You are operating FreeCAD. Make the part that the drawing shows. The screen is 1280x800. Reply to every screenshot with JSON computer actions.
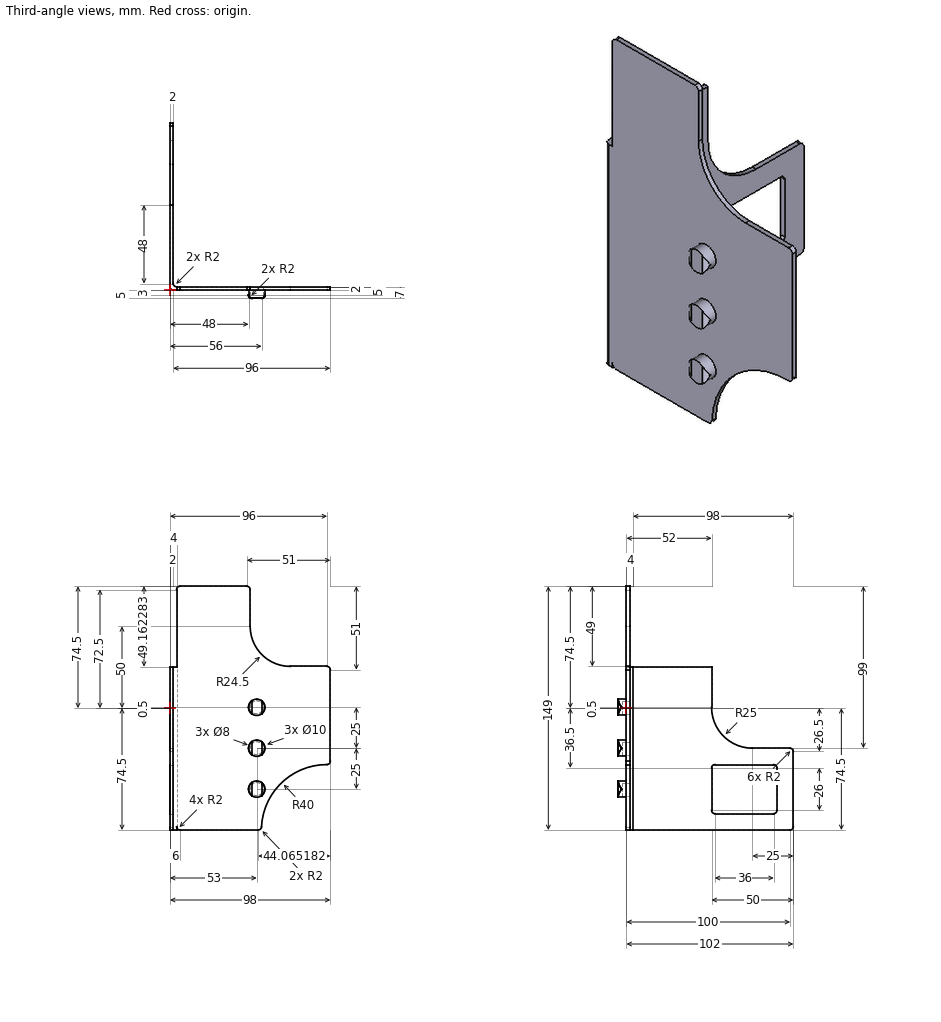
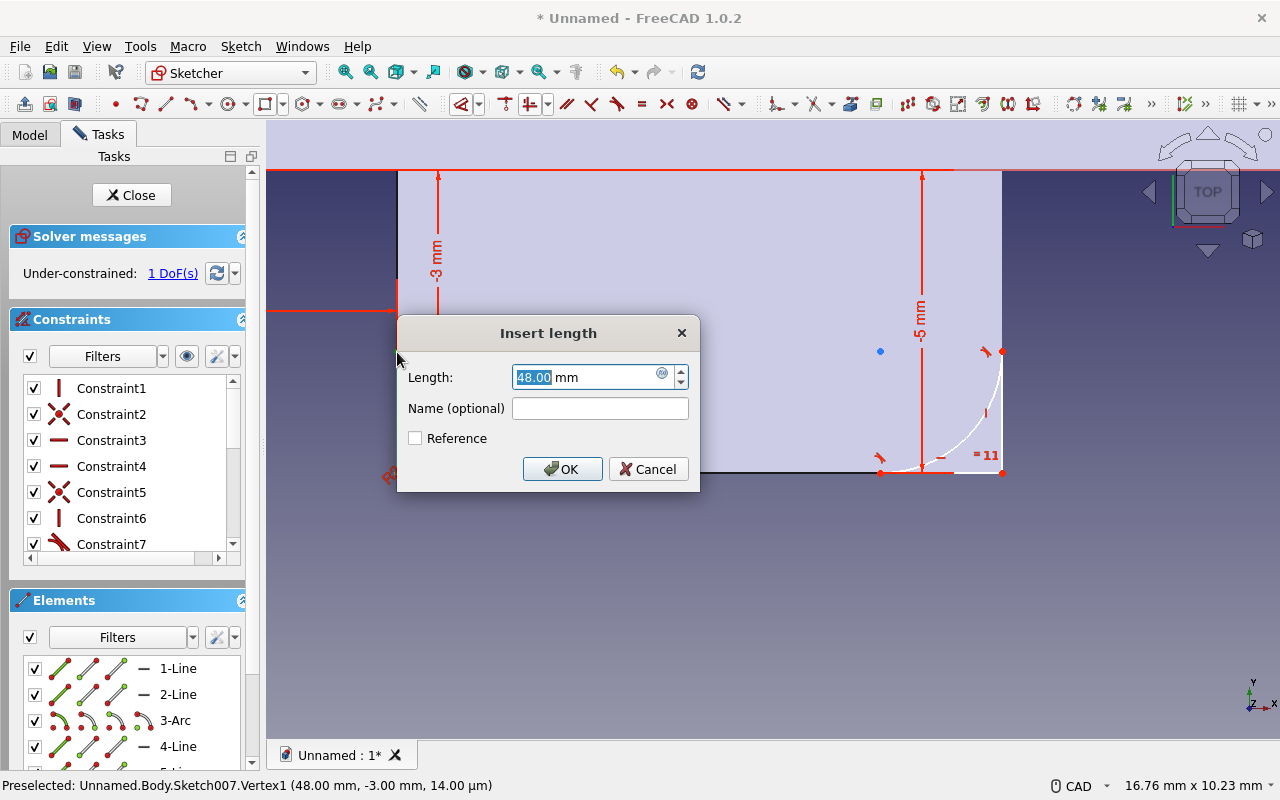
{"action": "type", "text": "48"}
{"action": "key", "text": "Return"}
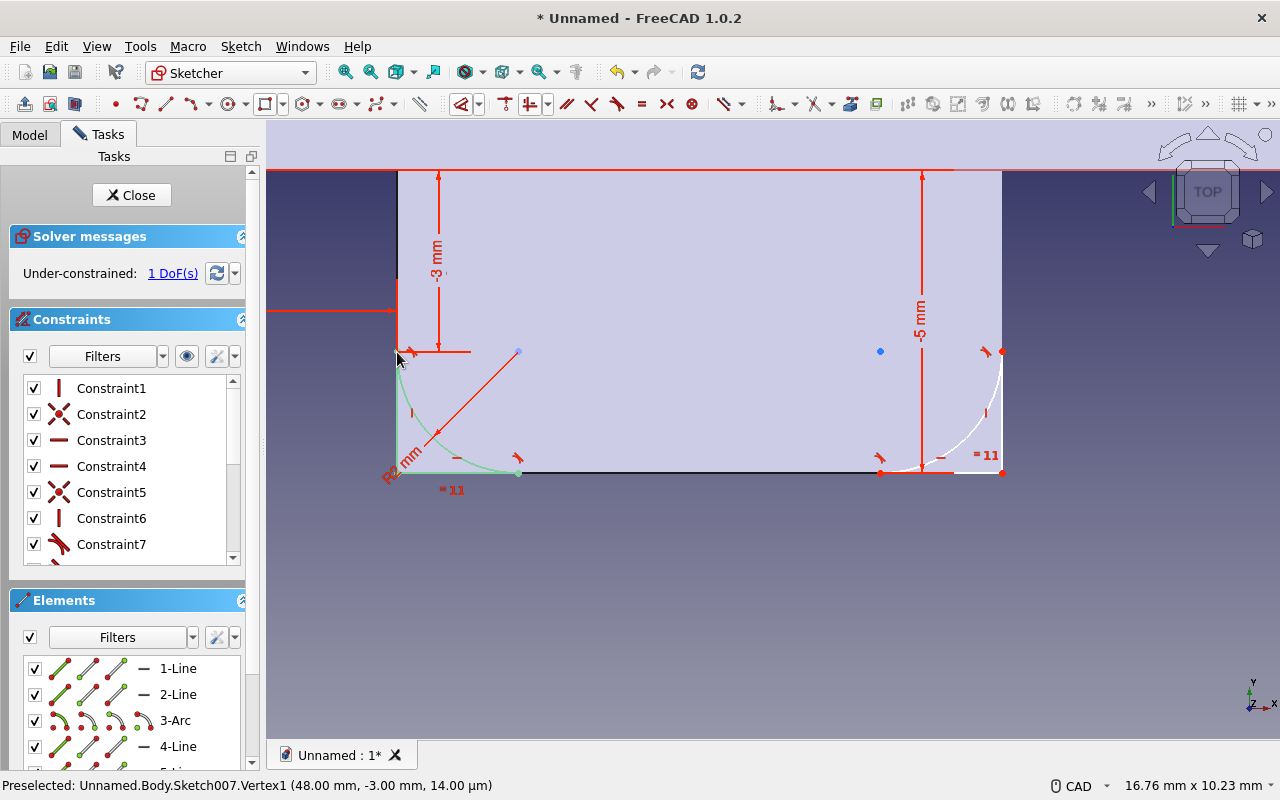
{"action": "left_click", "coordinate": [881, 473]}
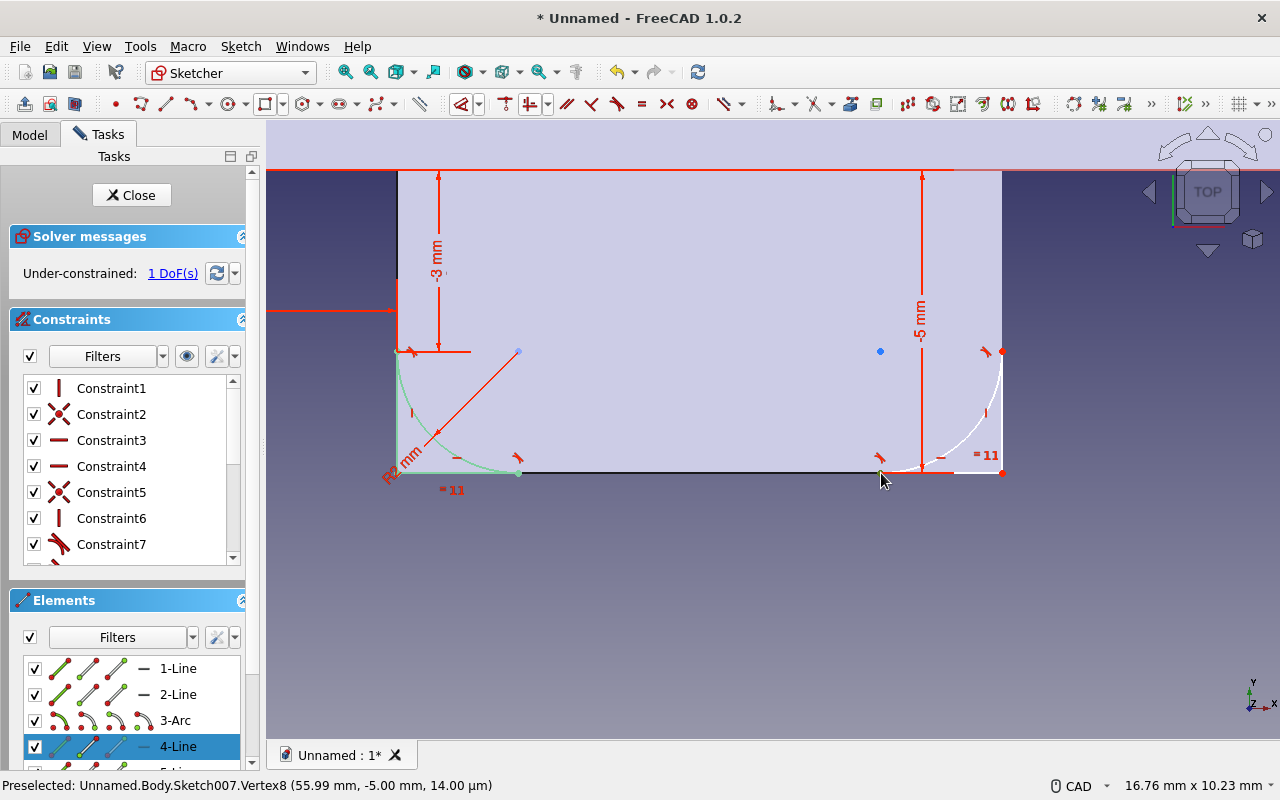
{"action": "key", "text": "l"}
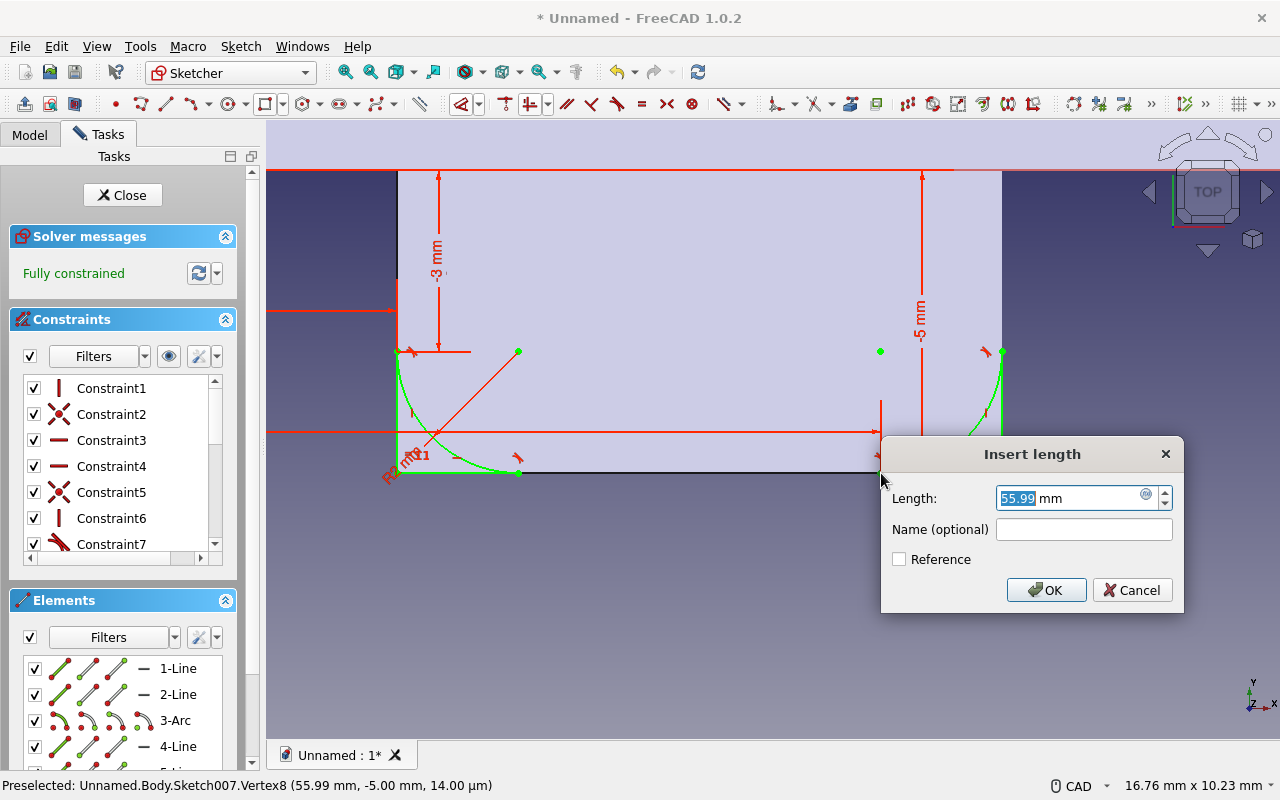
{"action": "type", "text": "56"}
{"action": "key", "text": "Return"}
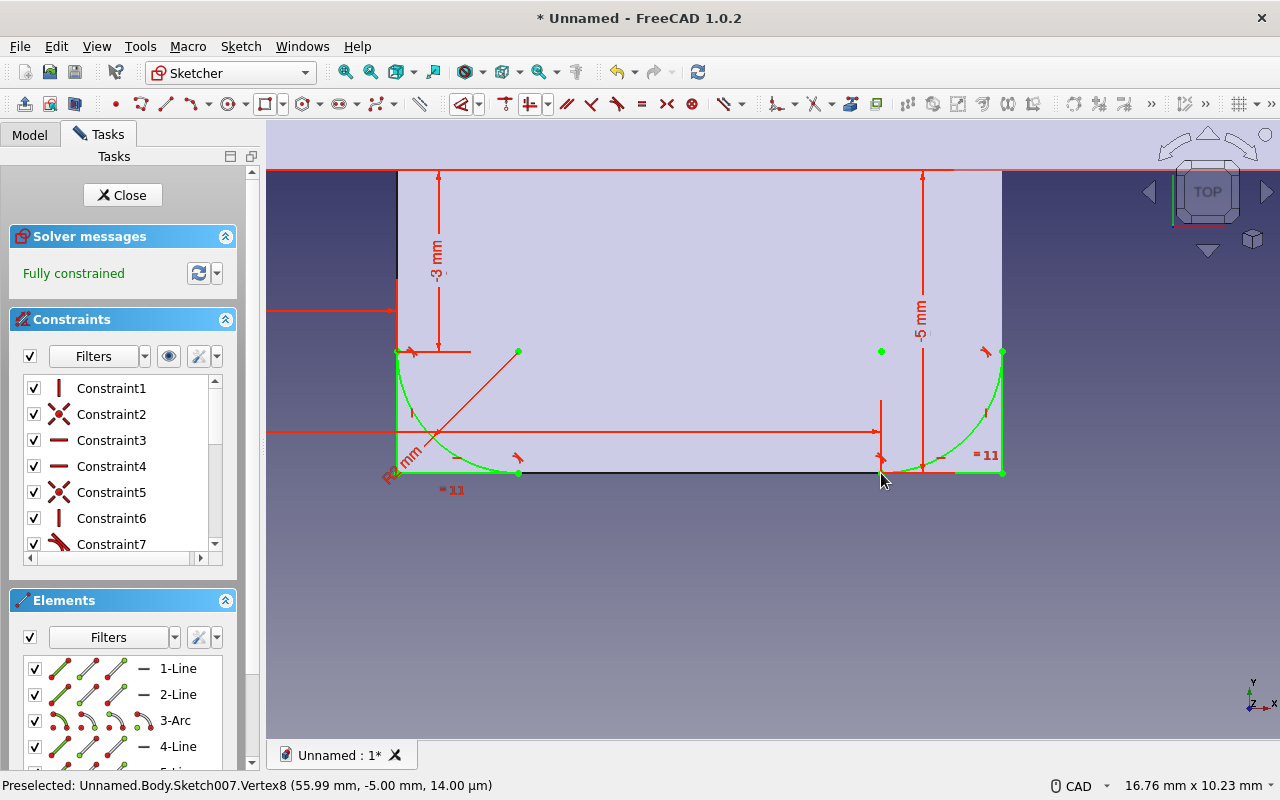
{"action": "left_click", "coordinate": [123, 195]}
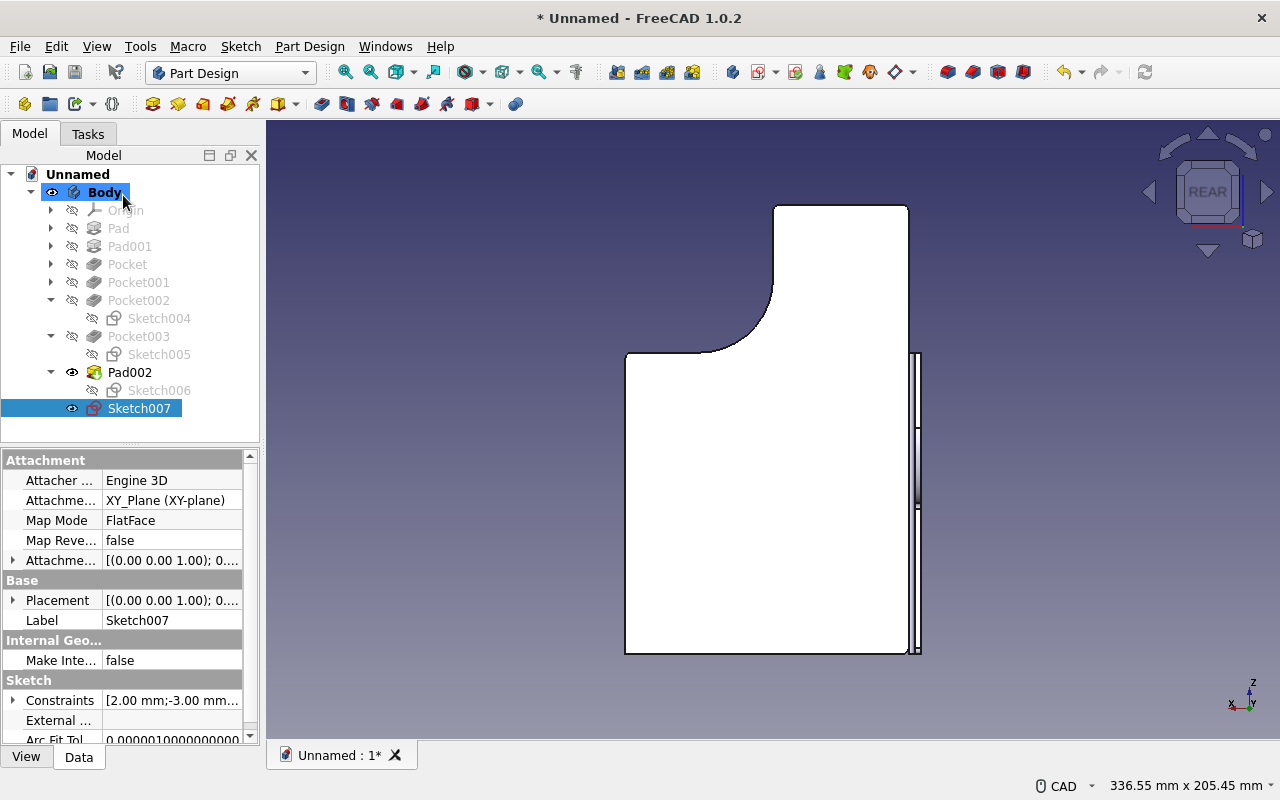
{"action": "left_click", "coordinate": [322, 104]}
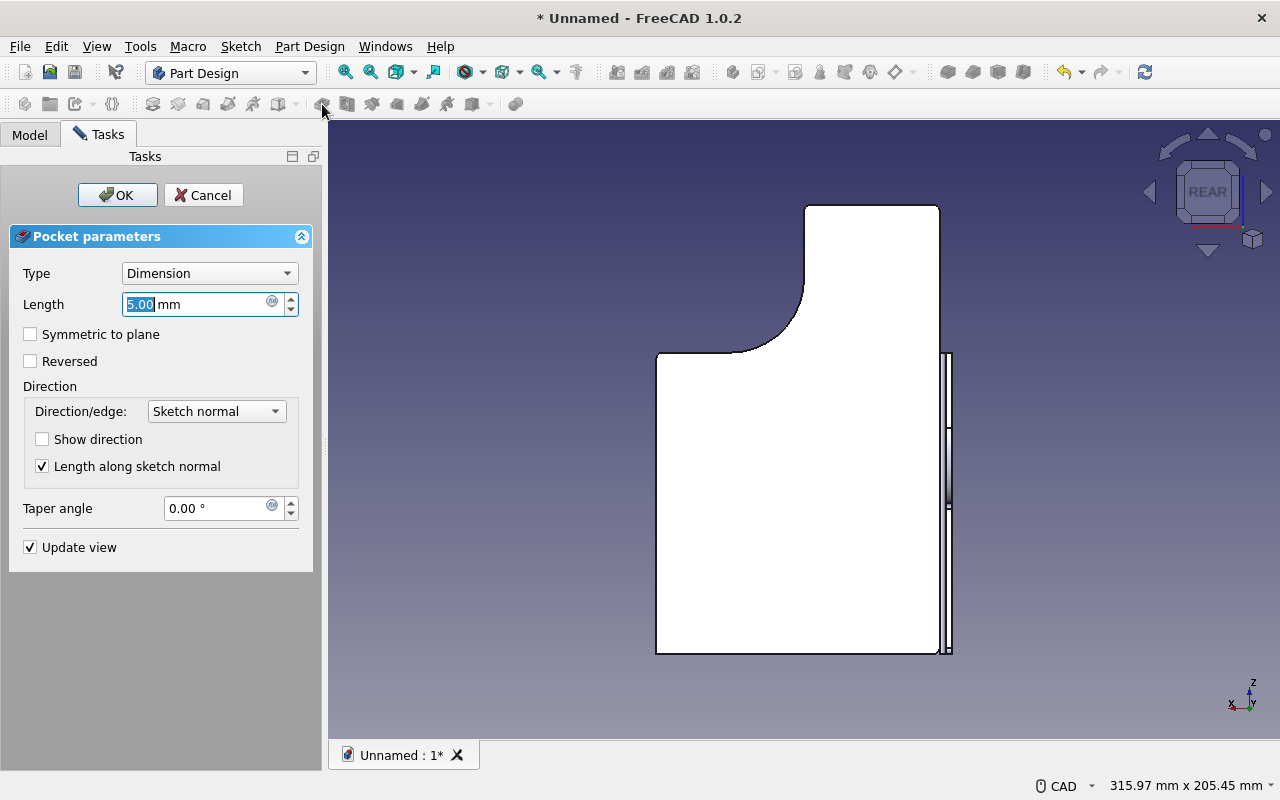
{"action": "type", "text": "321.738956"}
{"action": "key", "text": "Tab"}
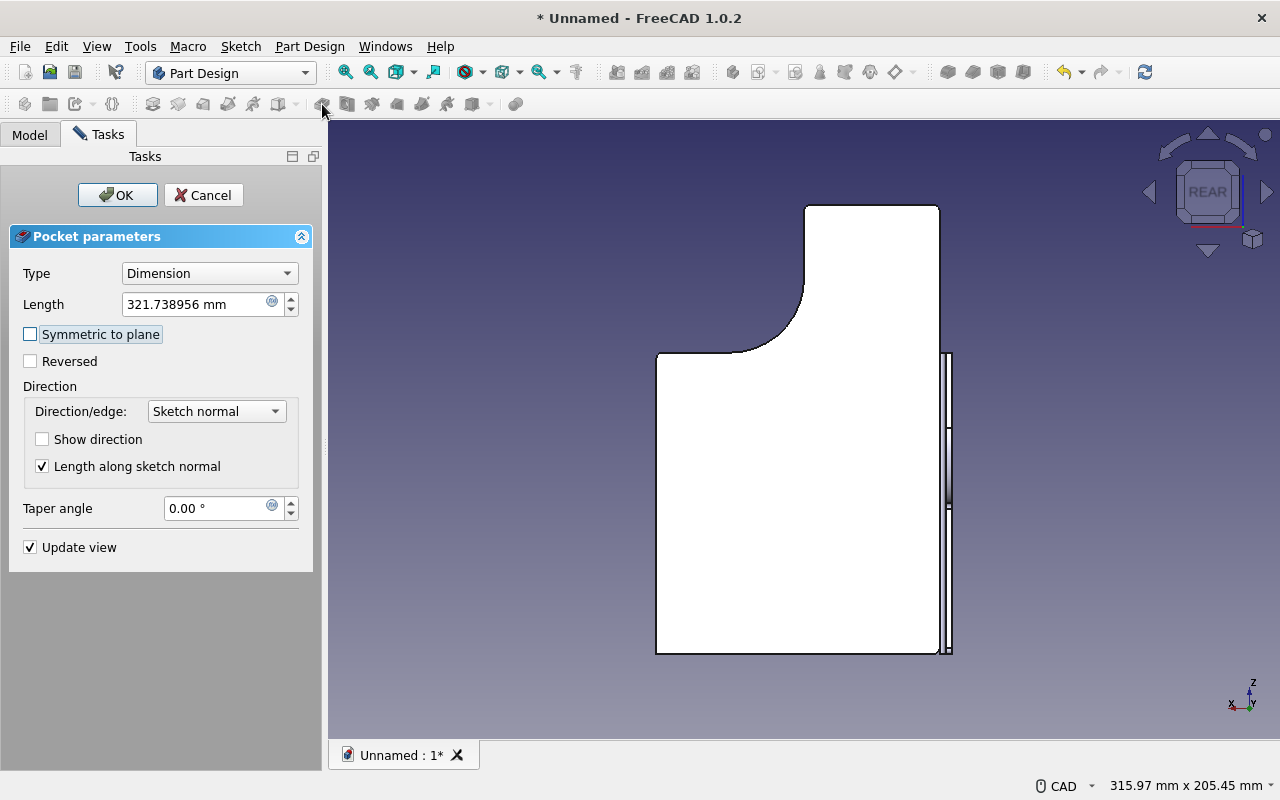
{"action": "left_click", "coordinate": [31, 334]}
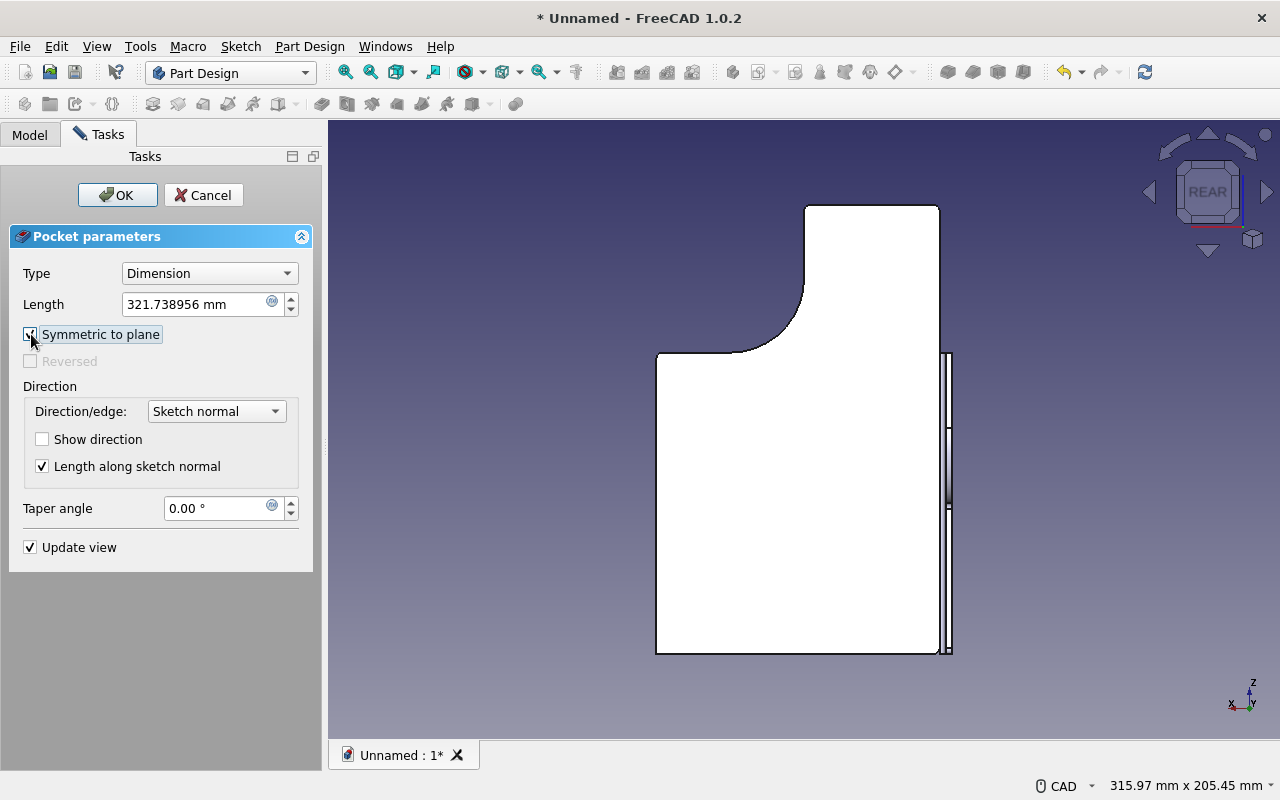
{"action": "left_click", "coordinate": [118, 195]}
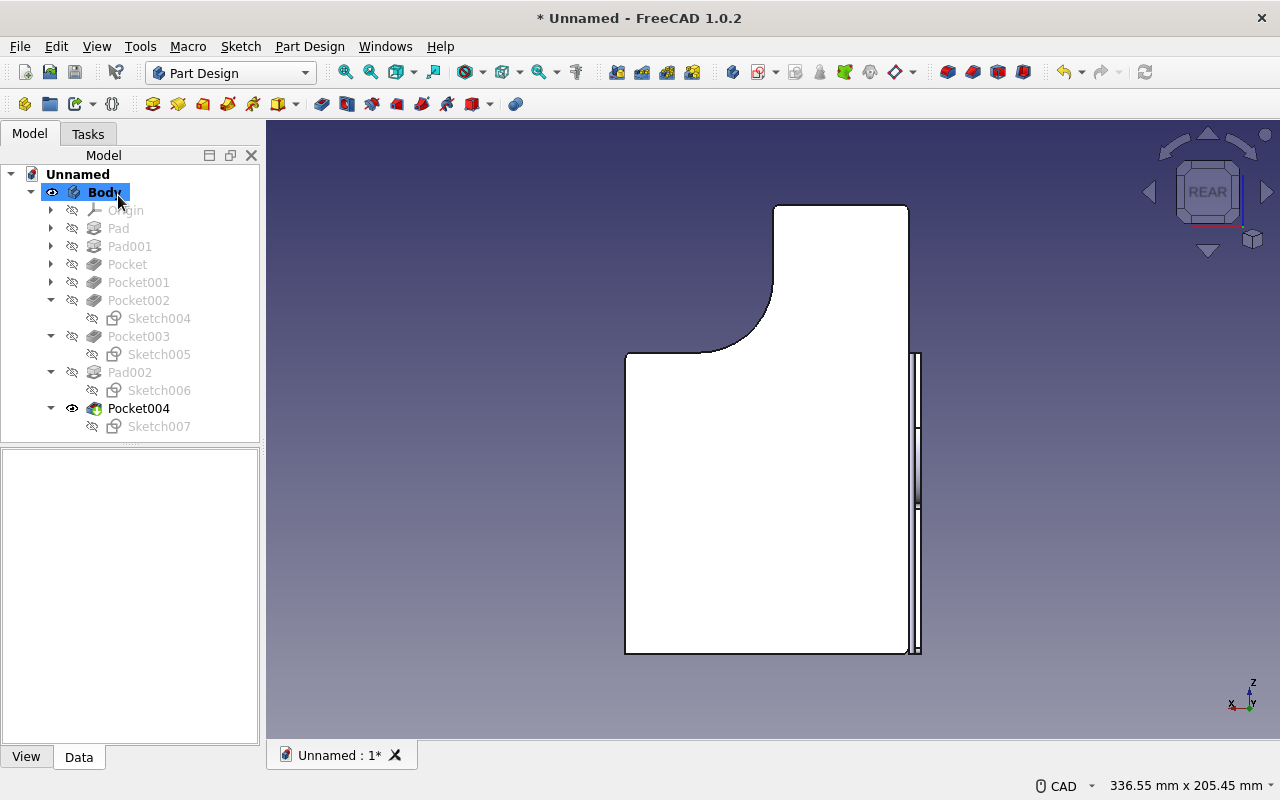
{"action": "left_click", "coordinate": [767, 493]}